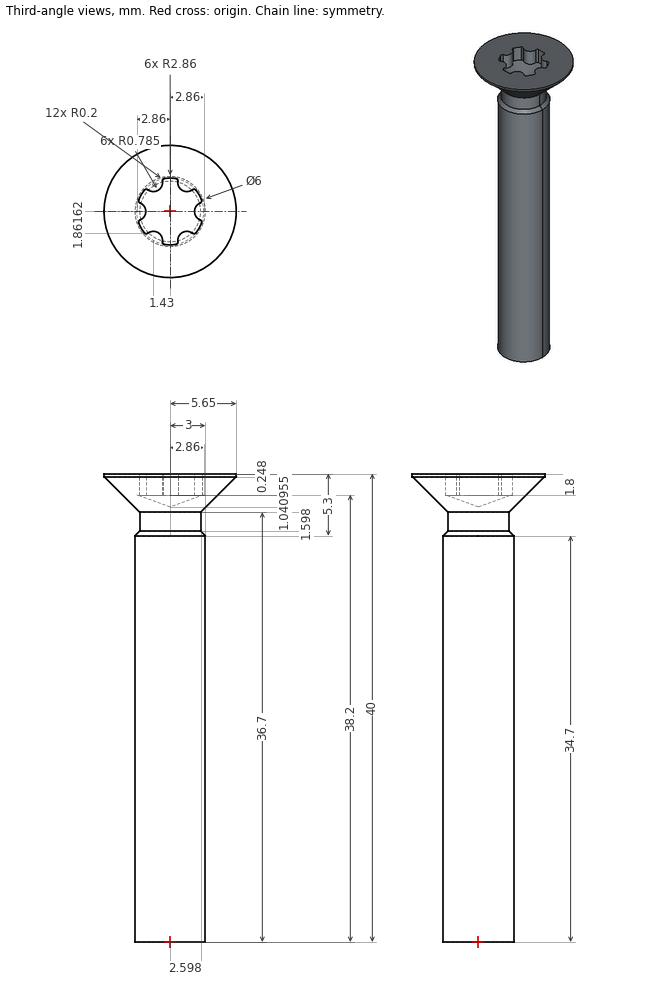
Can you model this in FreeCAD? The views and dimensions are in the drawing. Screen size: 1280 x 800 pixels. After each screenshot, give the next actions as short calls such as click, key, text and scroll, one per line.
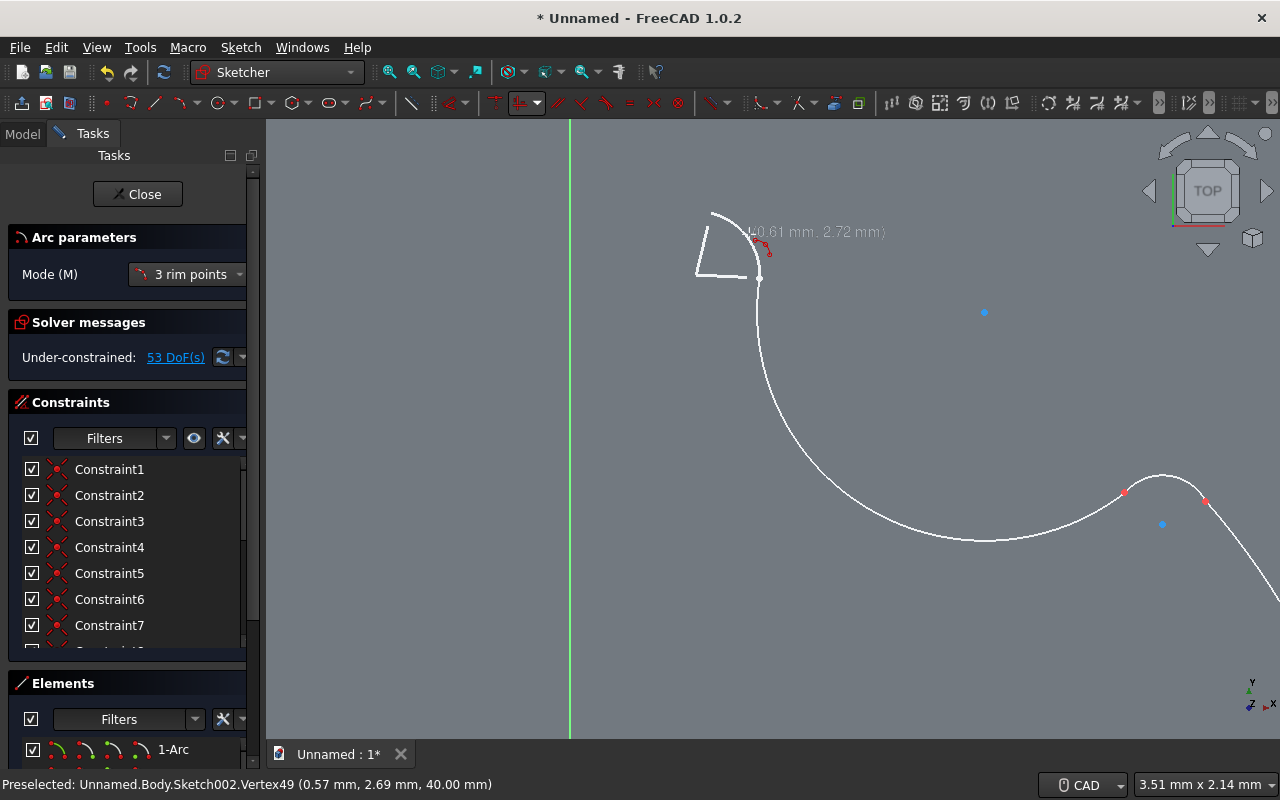
click(749, 234)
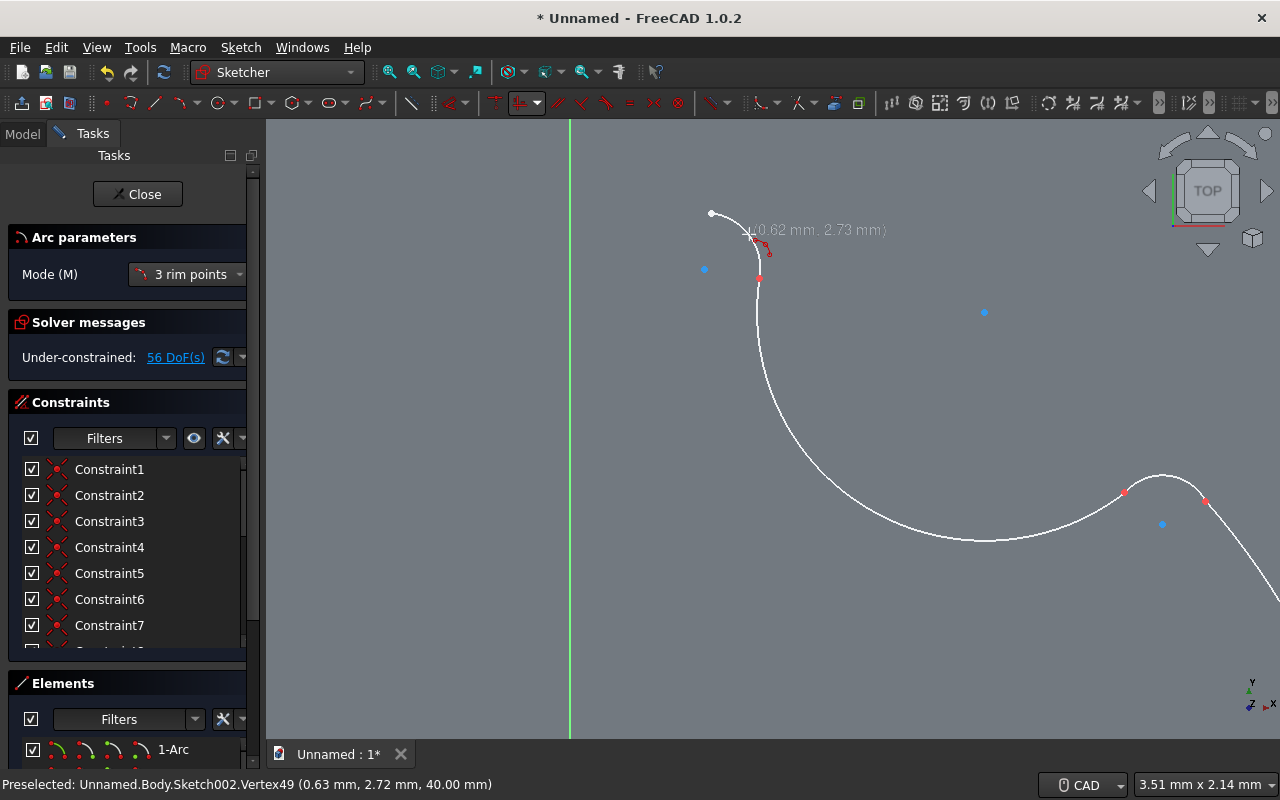
scroll(748, 234, down, 7)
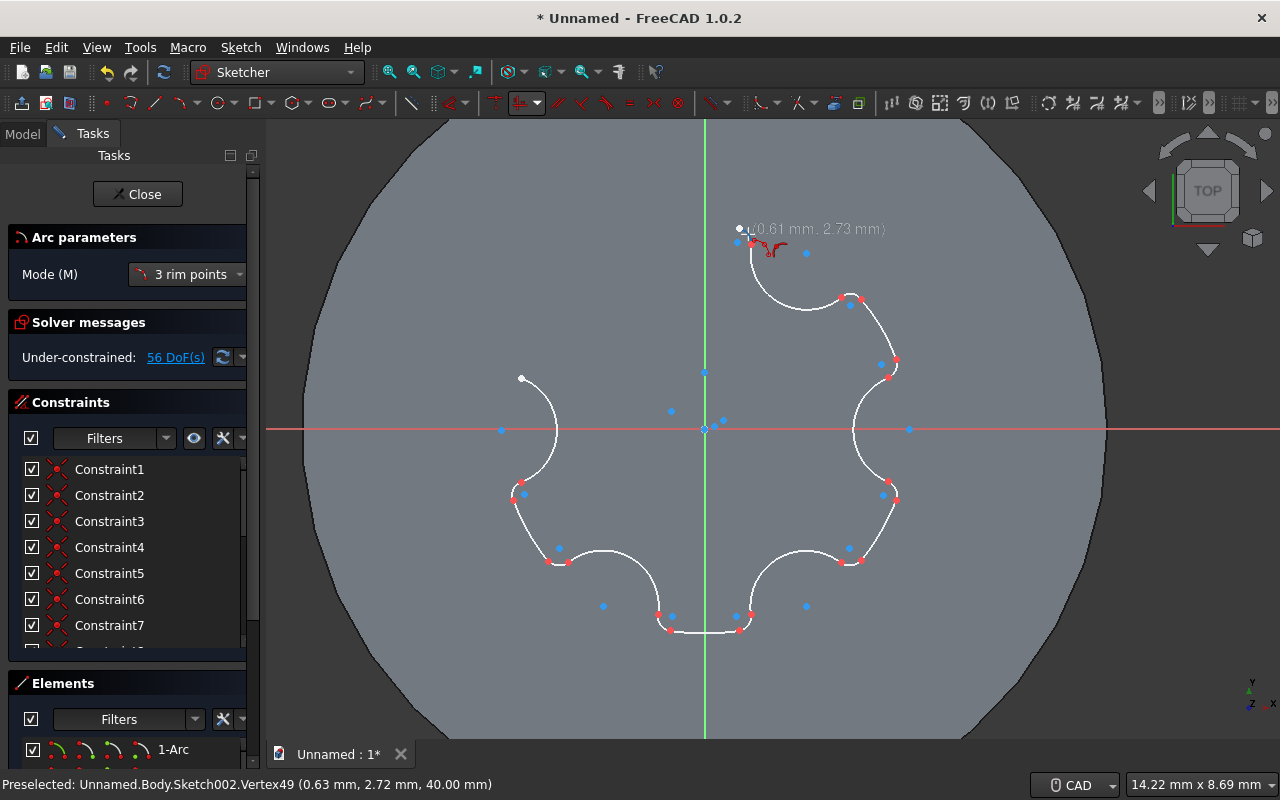
click(739, 229)
click(670, 228)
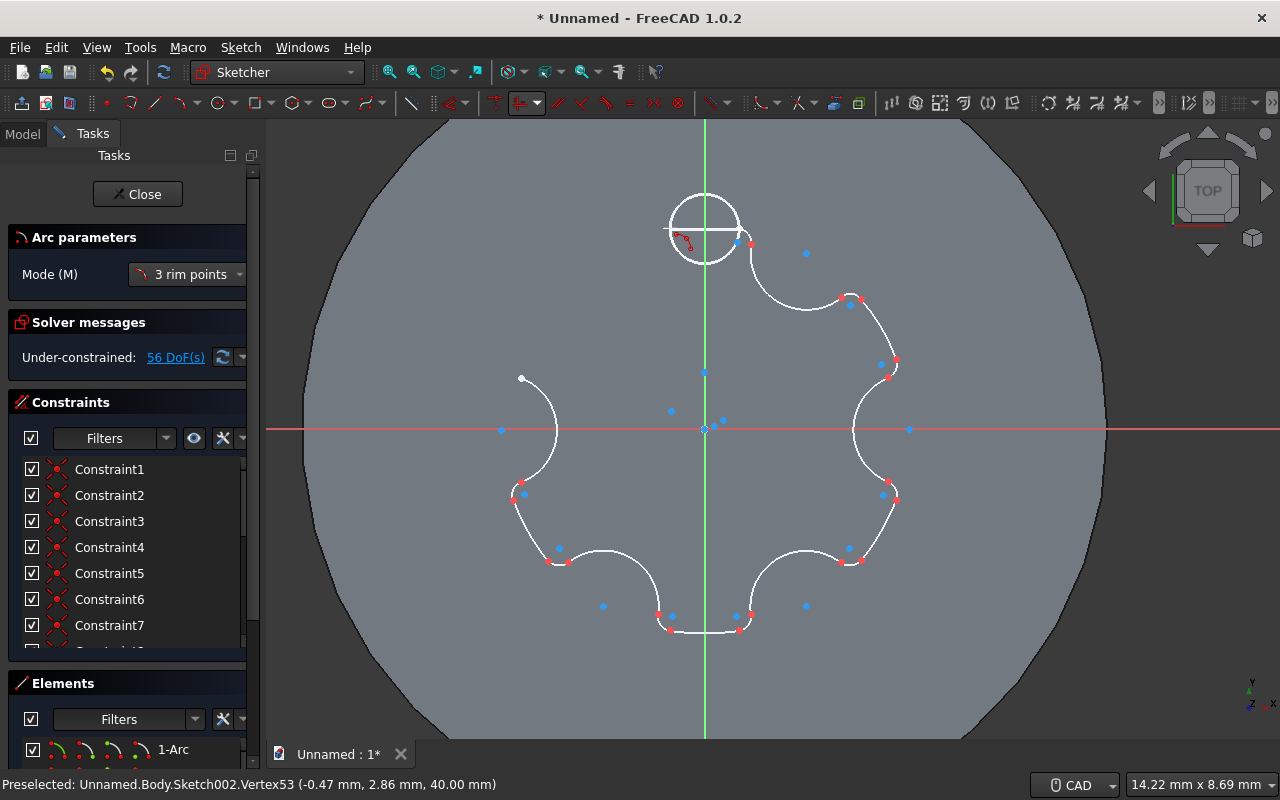
scroll(712, 225, up, 9)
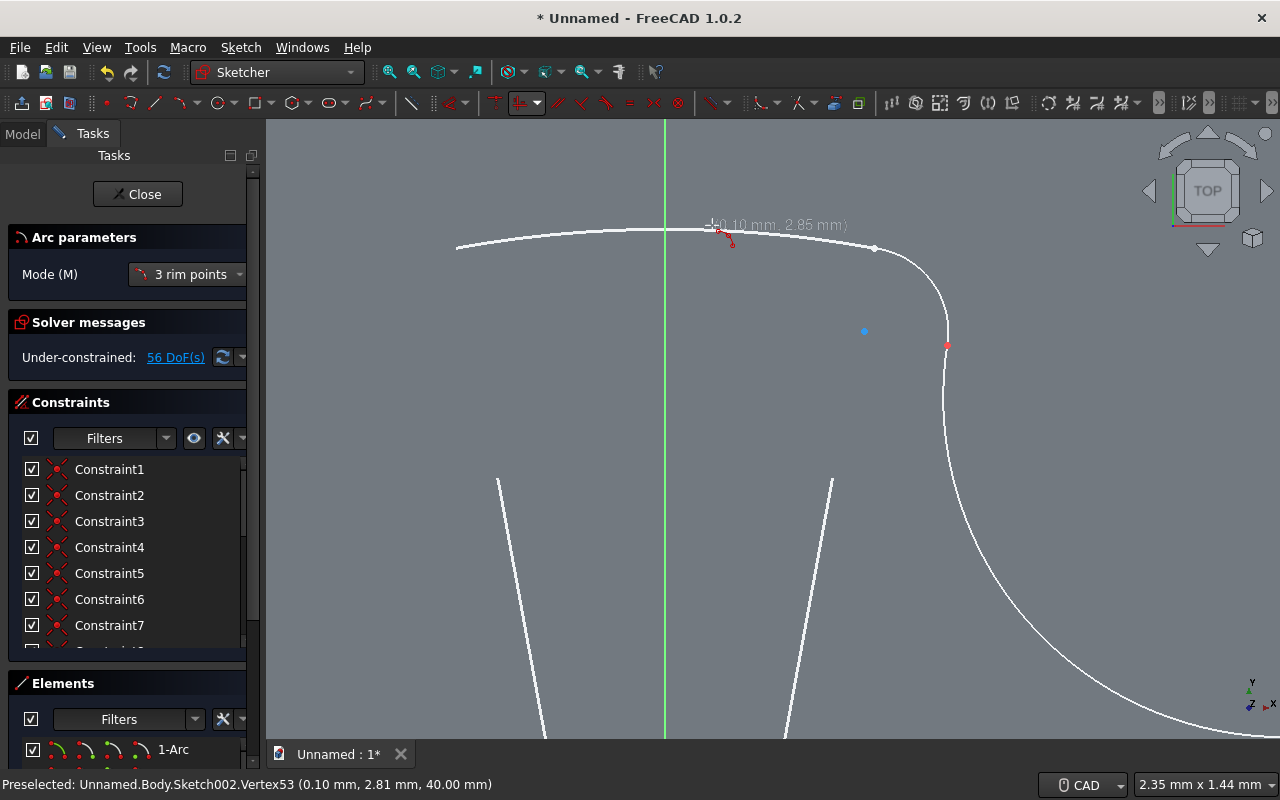
click(707, 227)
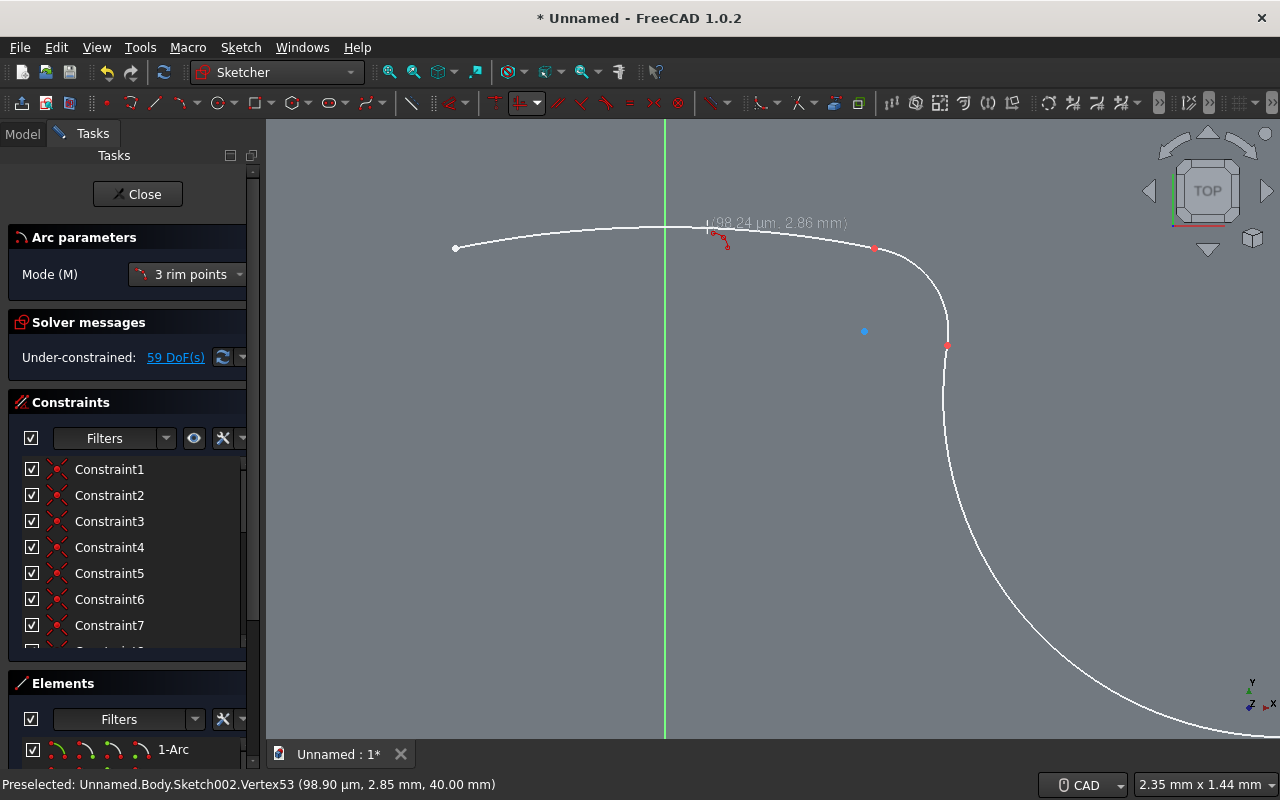
scroll(712, 225, down, 9)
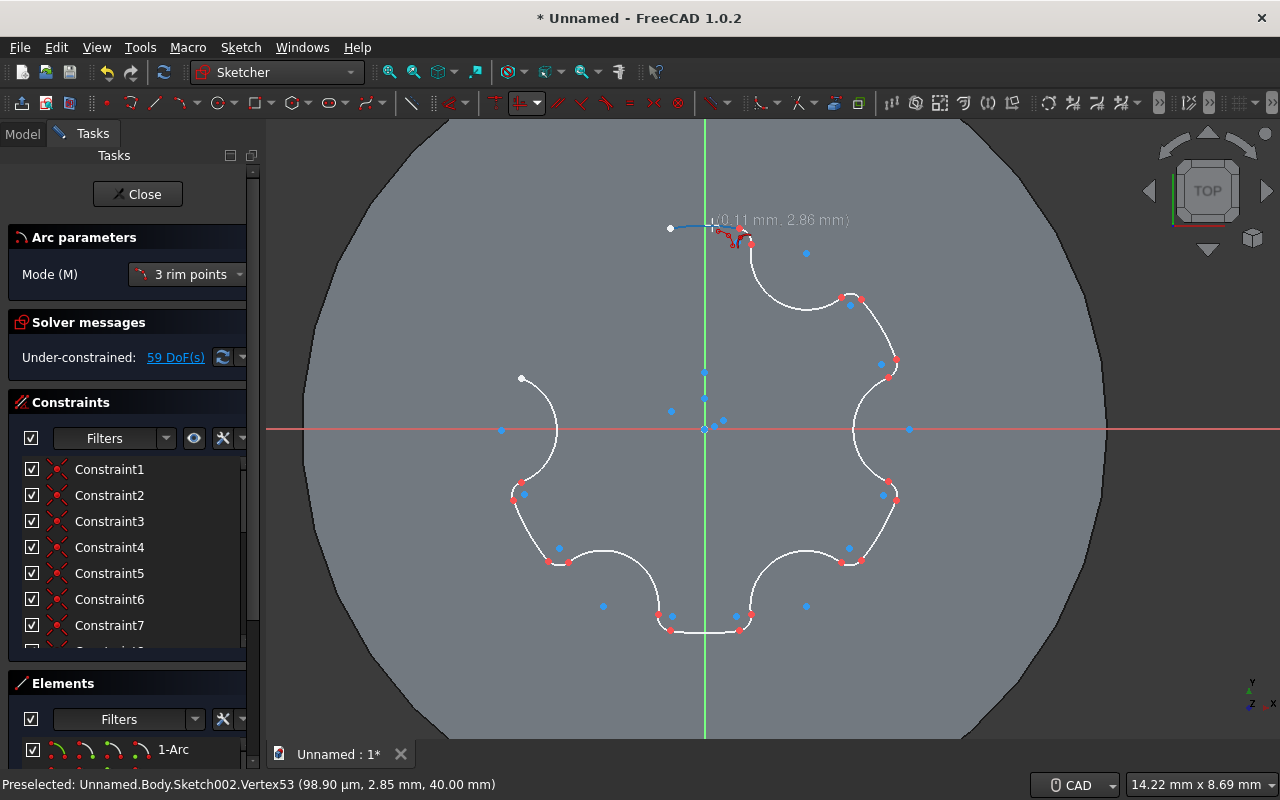
click(670, 229)
click(658, 244)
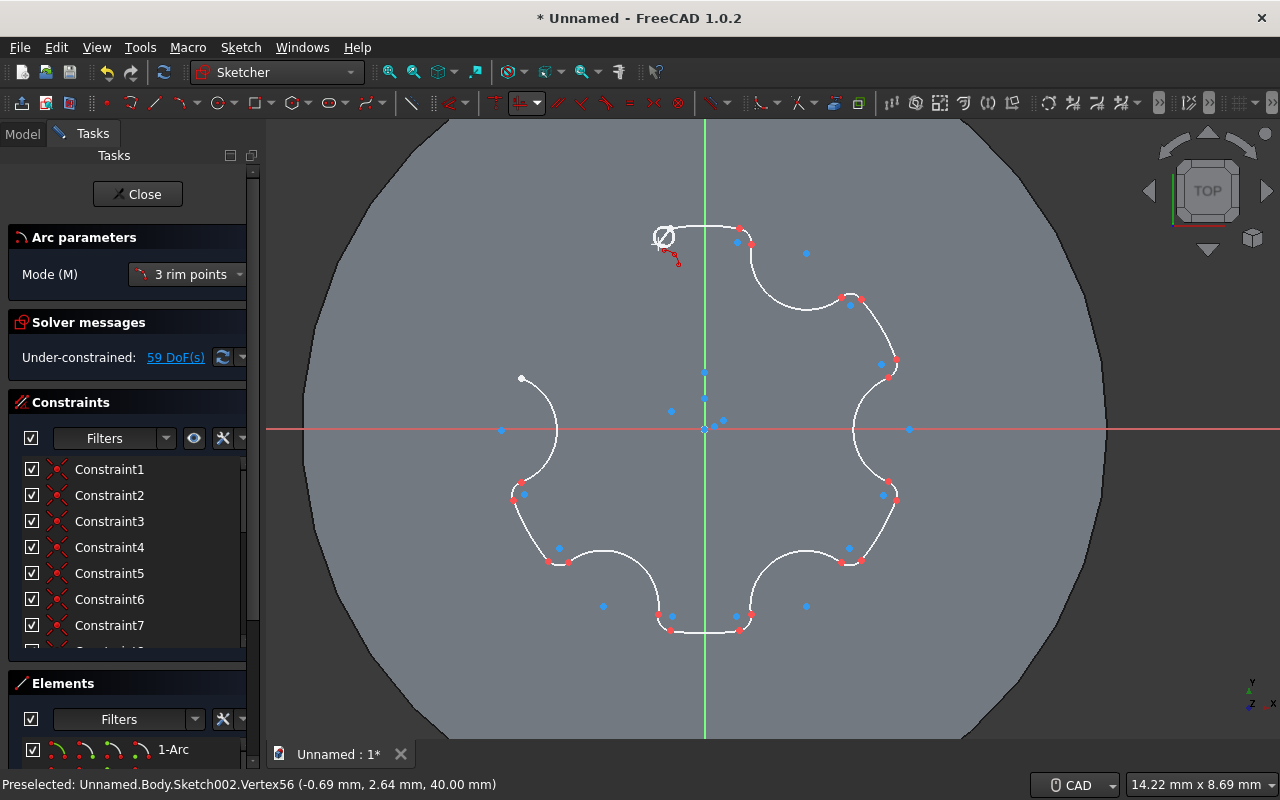
scroll(660, 234, up, 7)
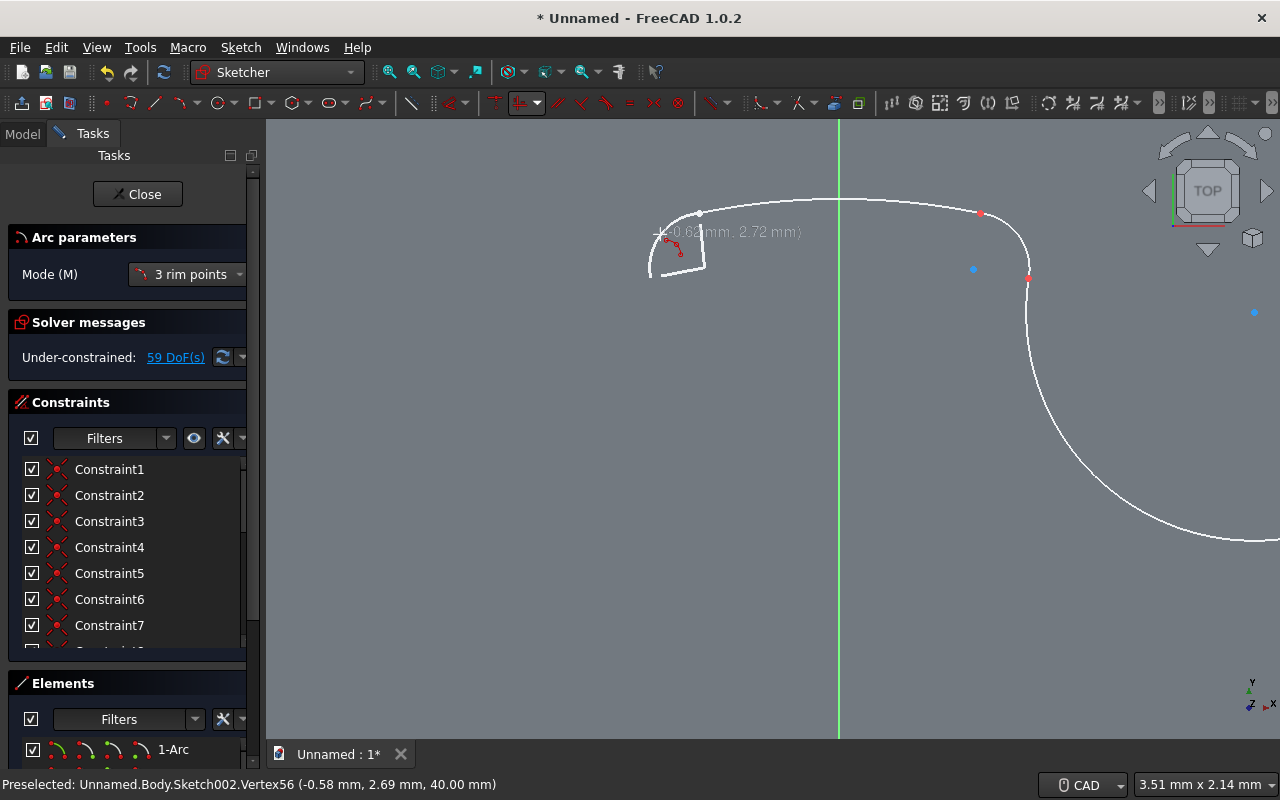
click(661, 234)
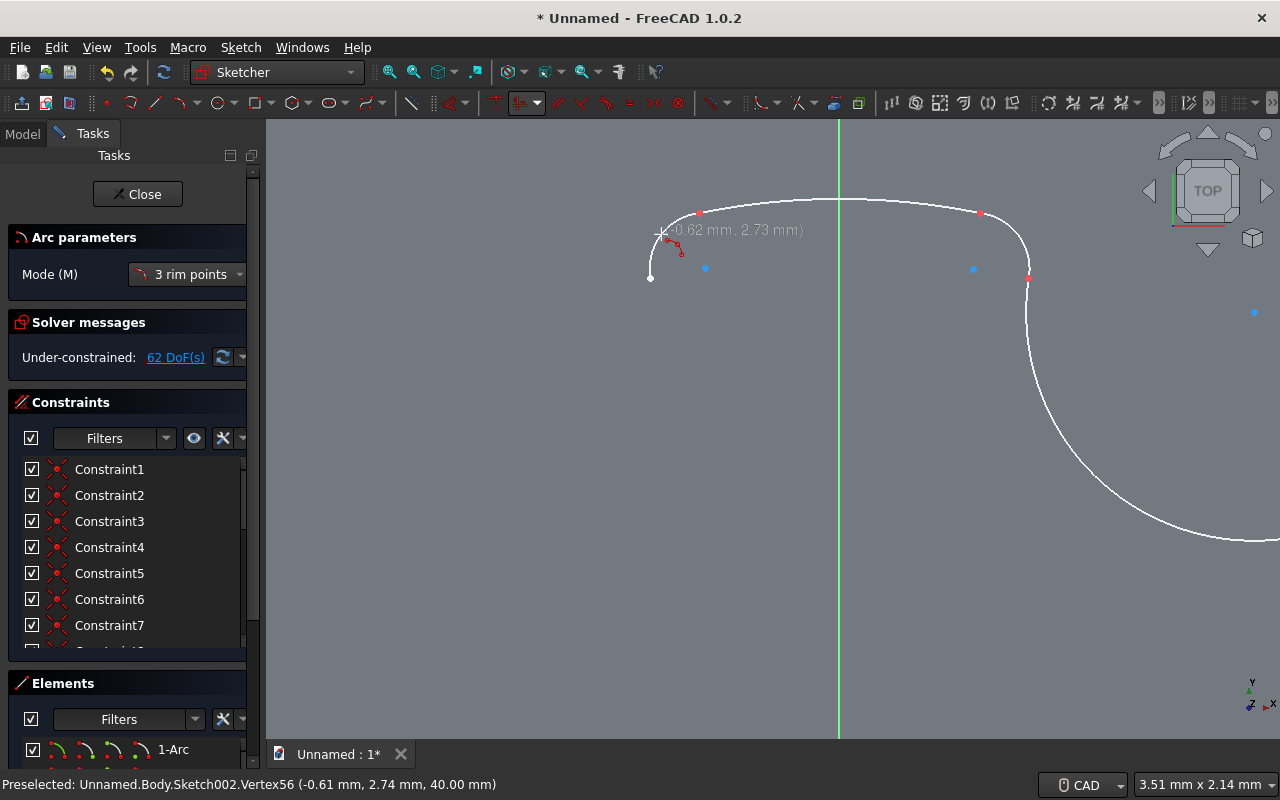
scroll(660, 234, down, 7)